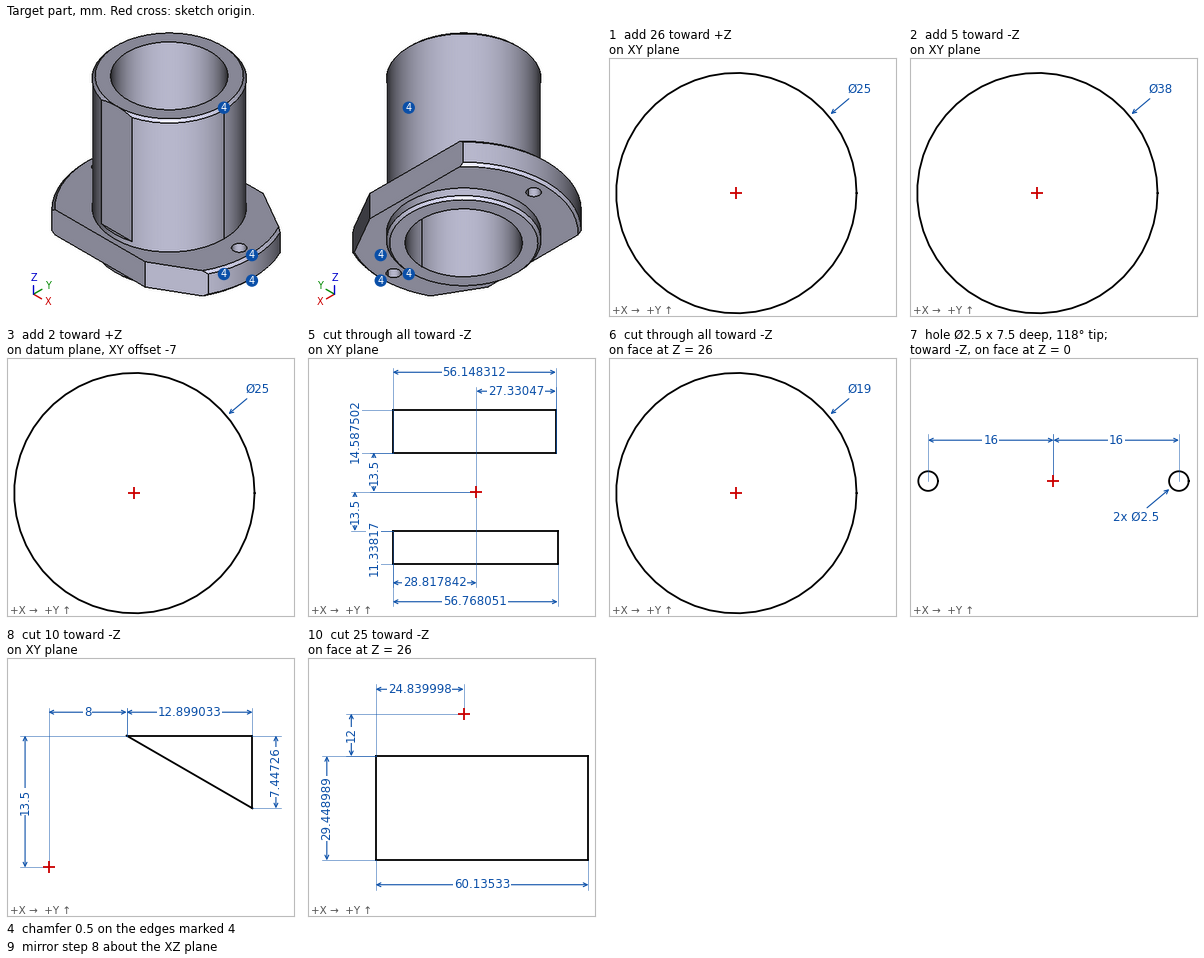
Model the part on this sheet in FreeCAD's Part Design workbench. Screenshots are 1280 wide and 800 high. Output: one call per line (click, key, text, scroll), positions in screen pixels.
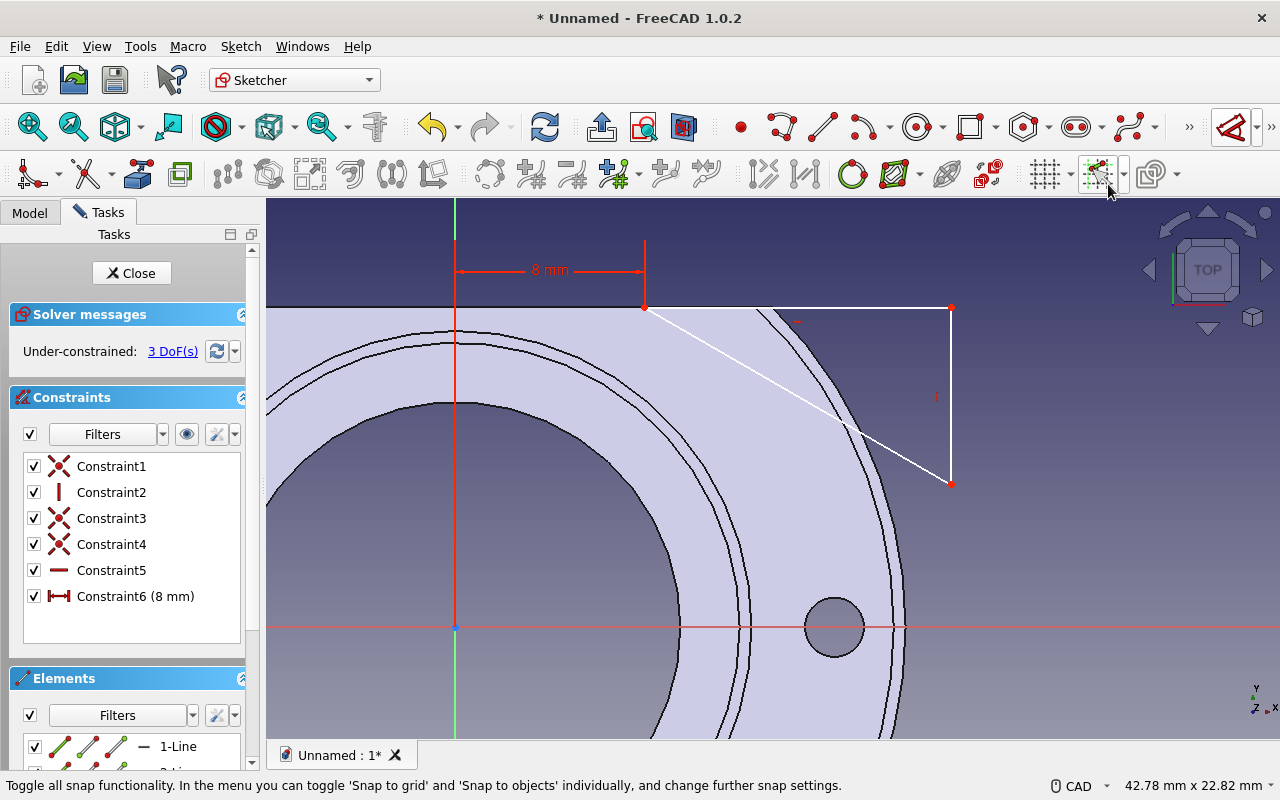
click(645, 308)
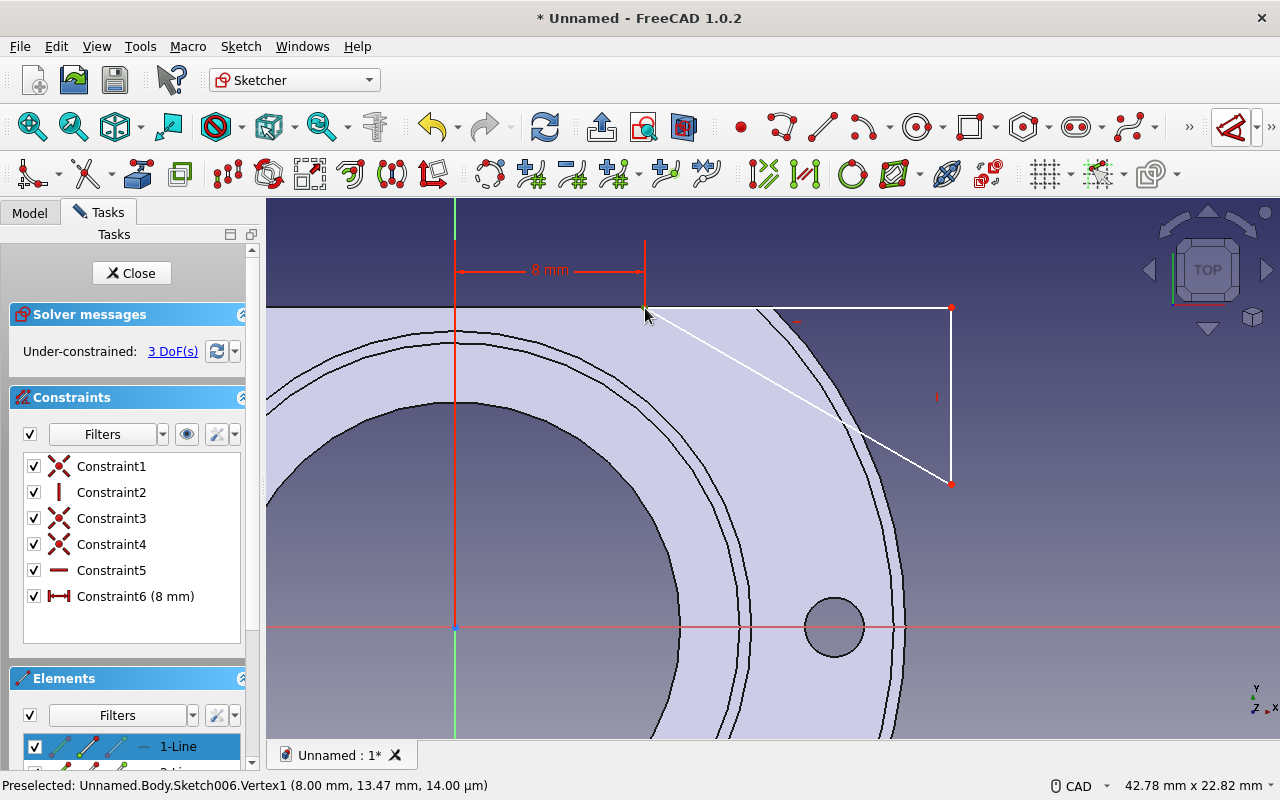
click(1256, 128)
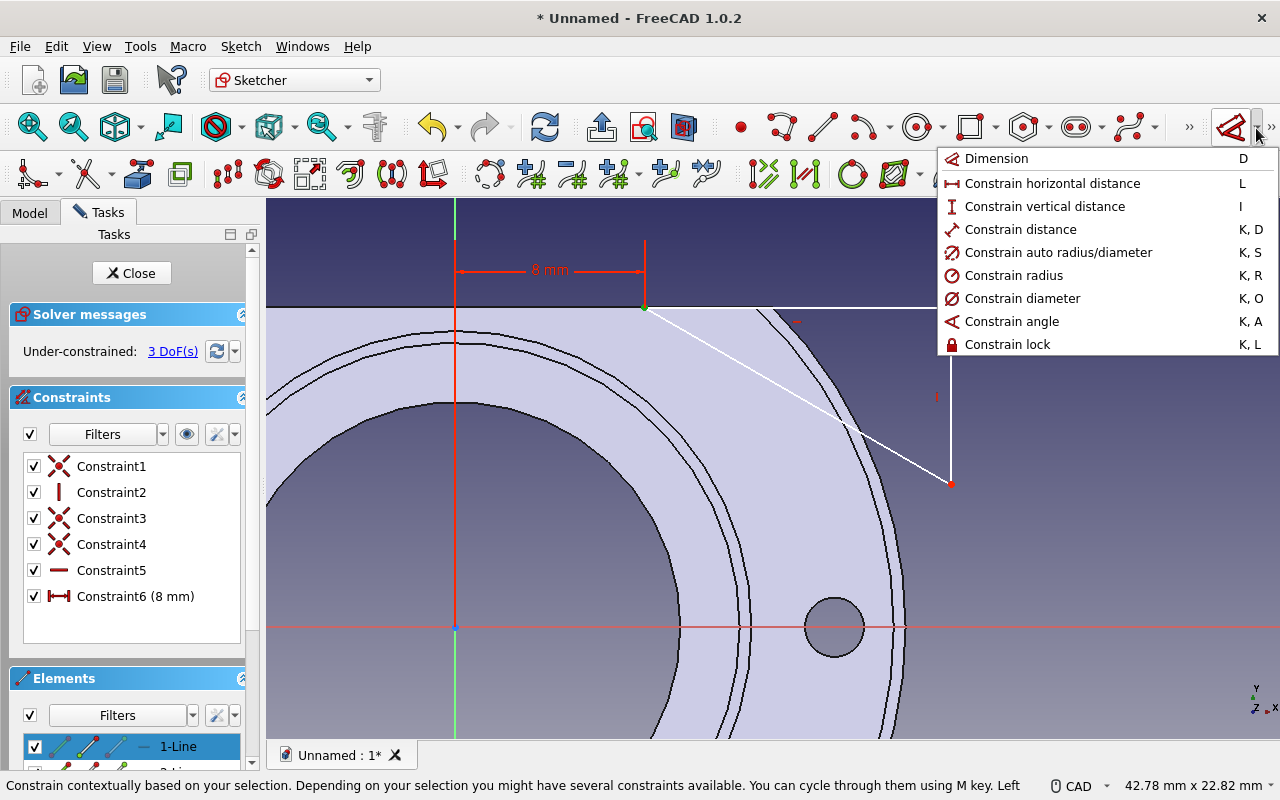
click(1108, 206)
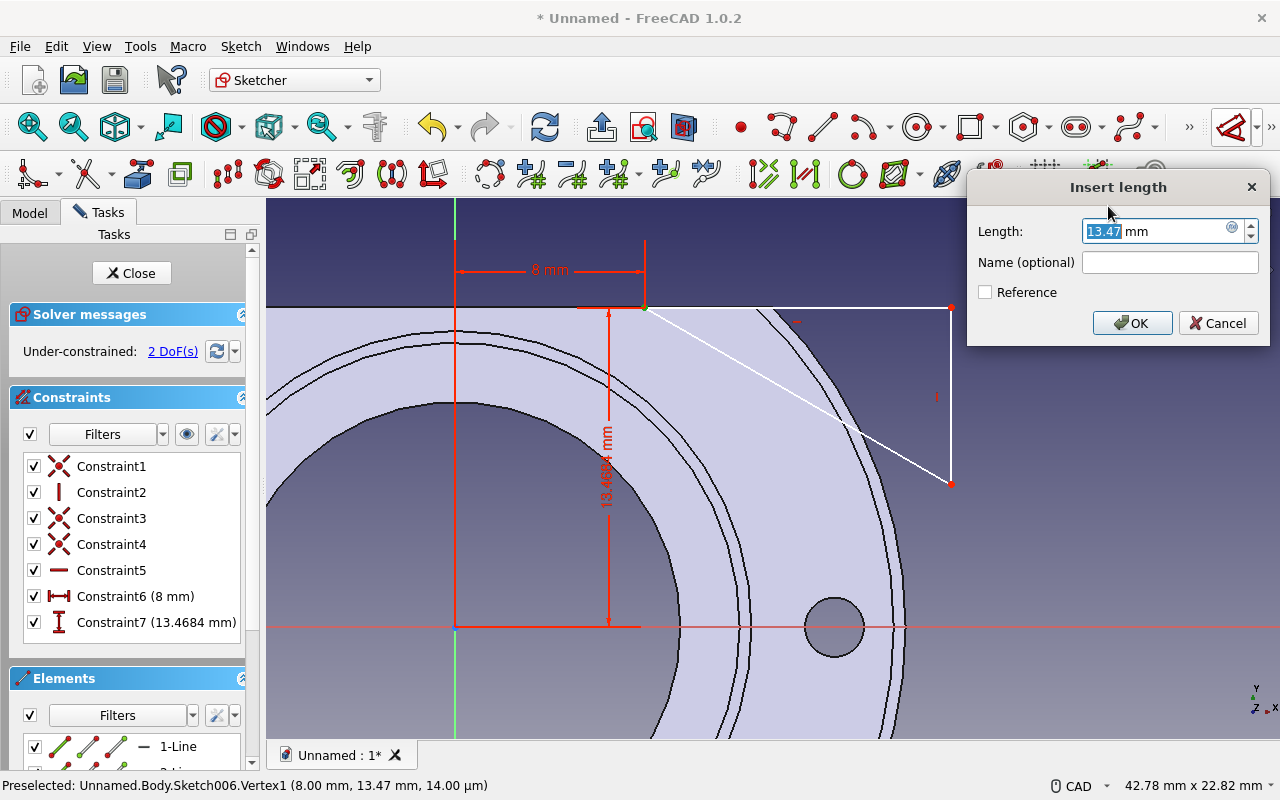
text(13.5)
key(Return)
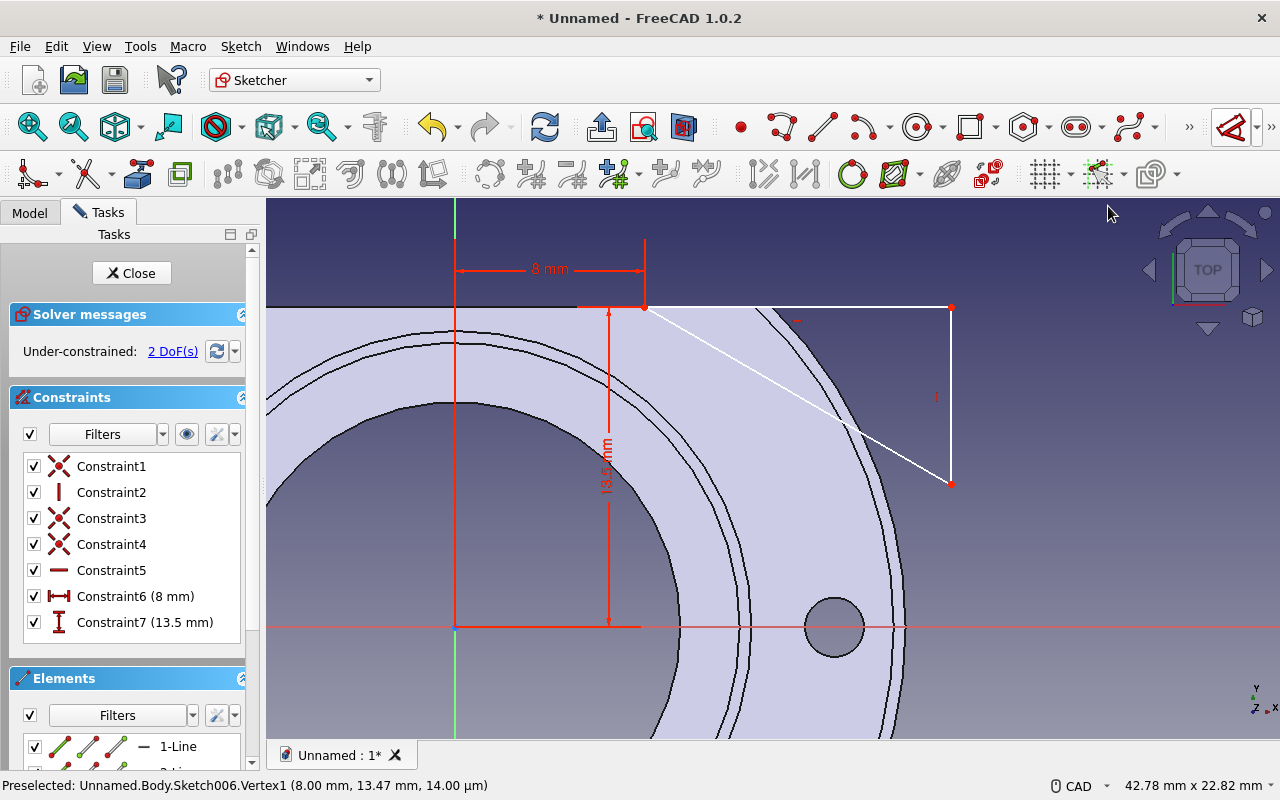
click(951, 432)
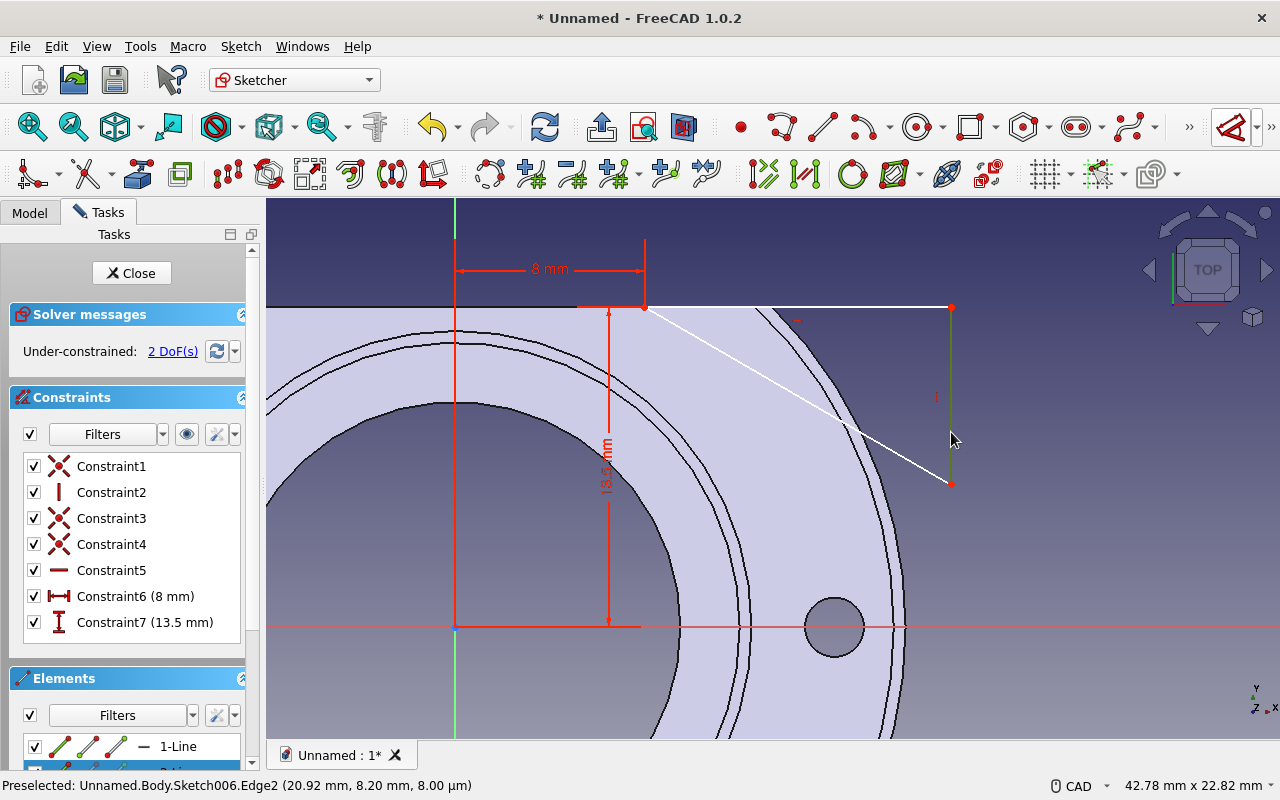
key(i)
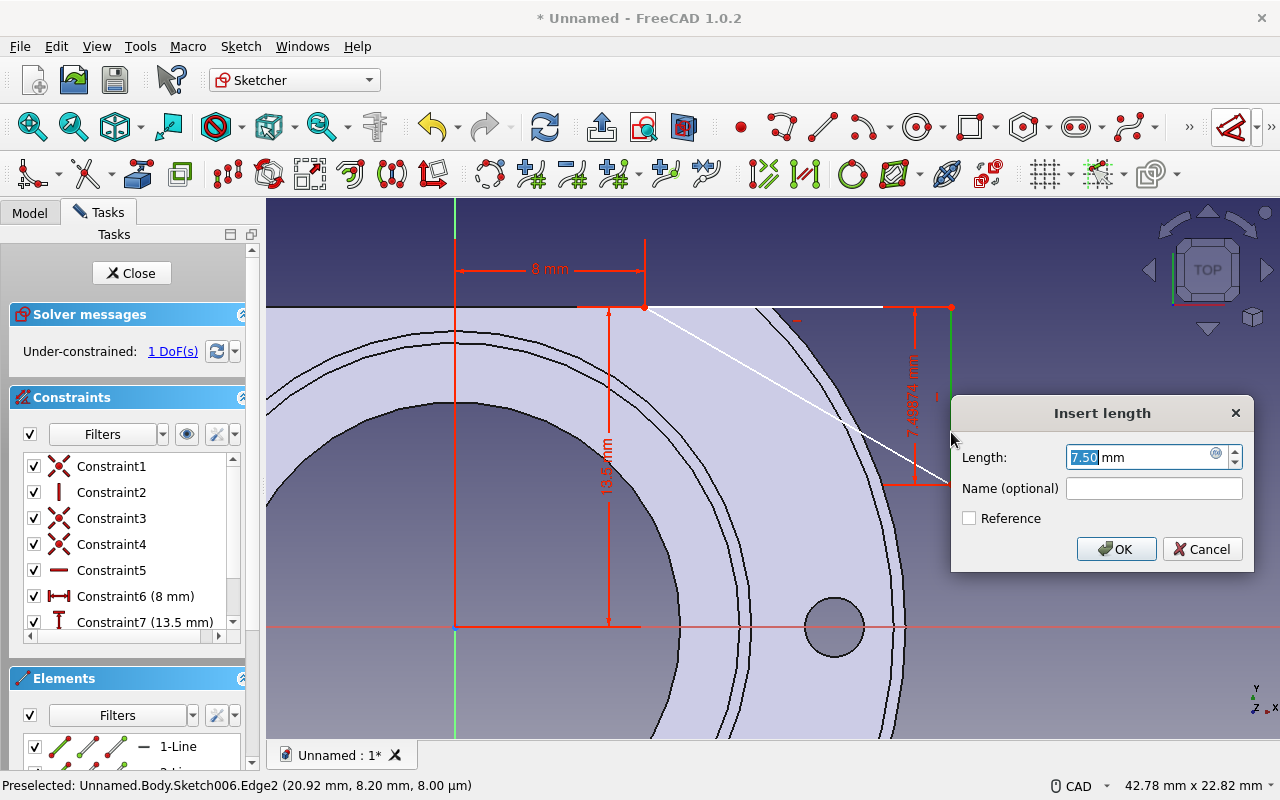
text(7.44726)
key(Return)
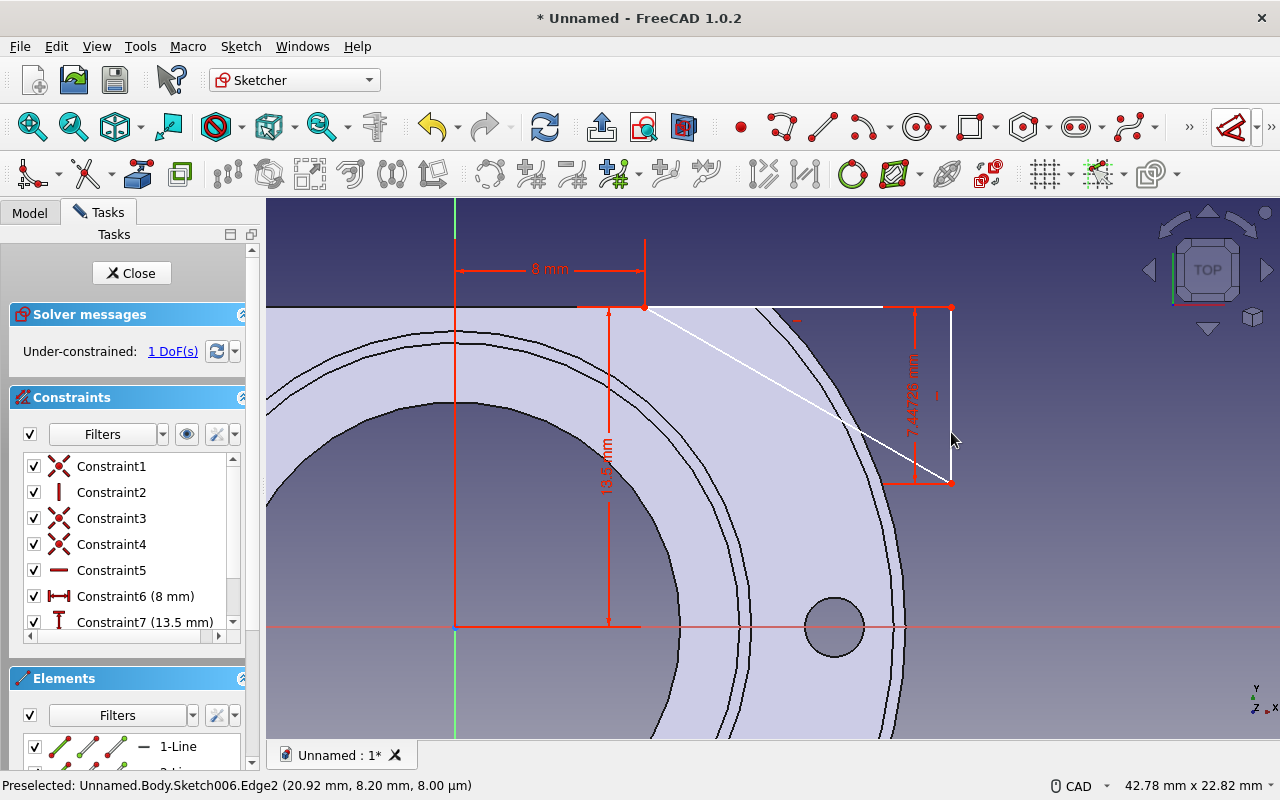
click(859, 307)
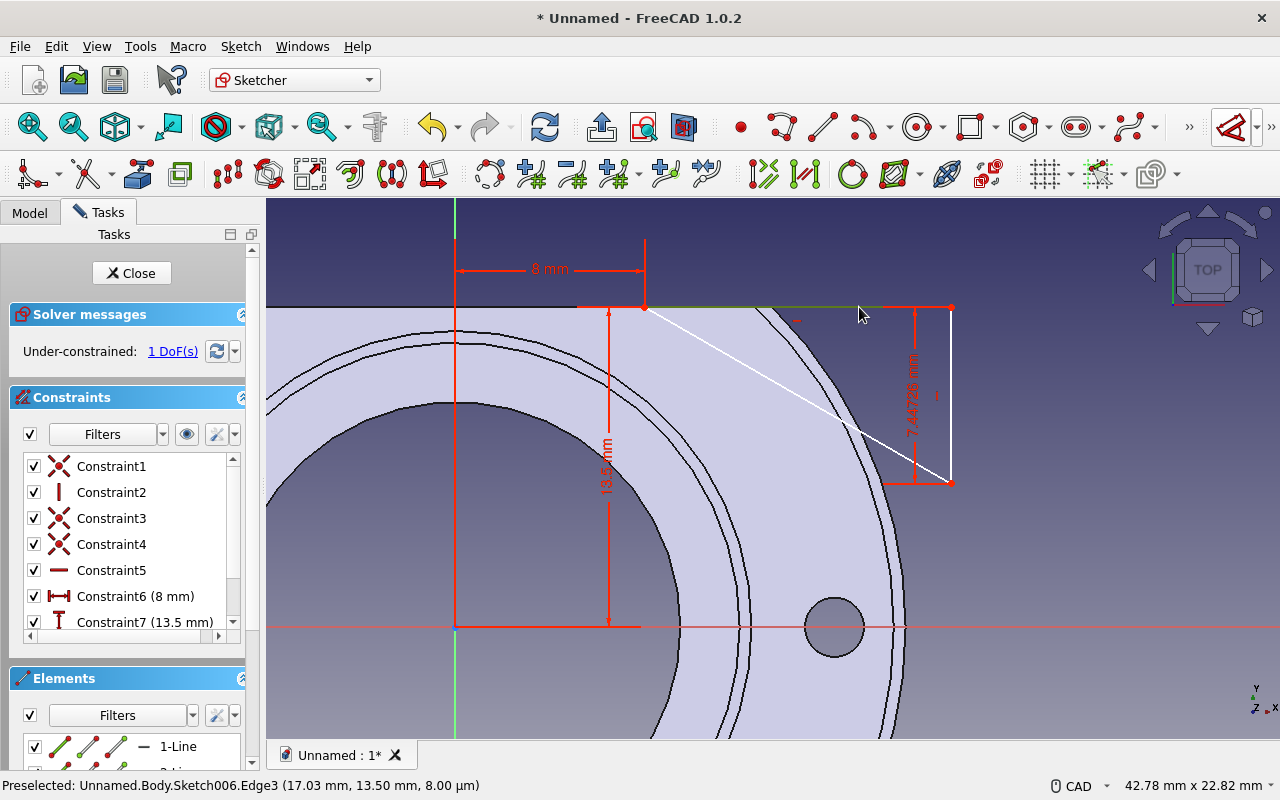
key(l)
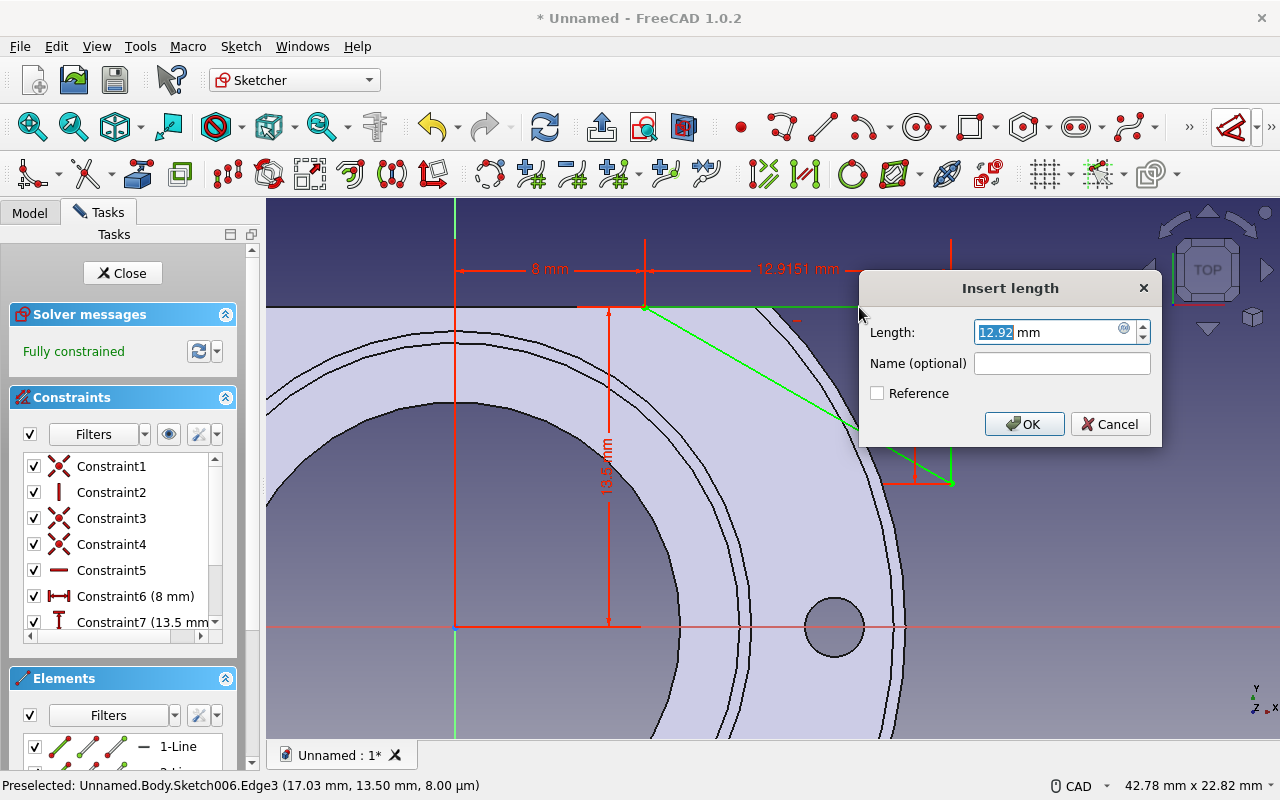
text(12.899033)
key(Return)